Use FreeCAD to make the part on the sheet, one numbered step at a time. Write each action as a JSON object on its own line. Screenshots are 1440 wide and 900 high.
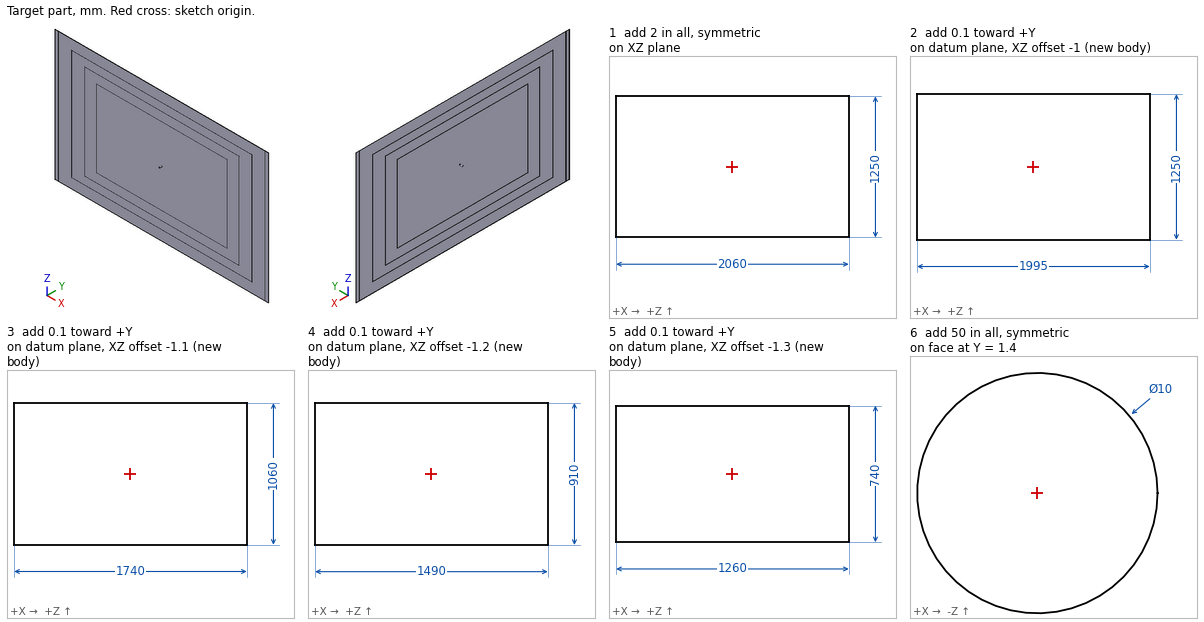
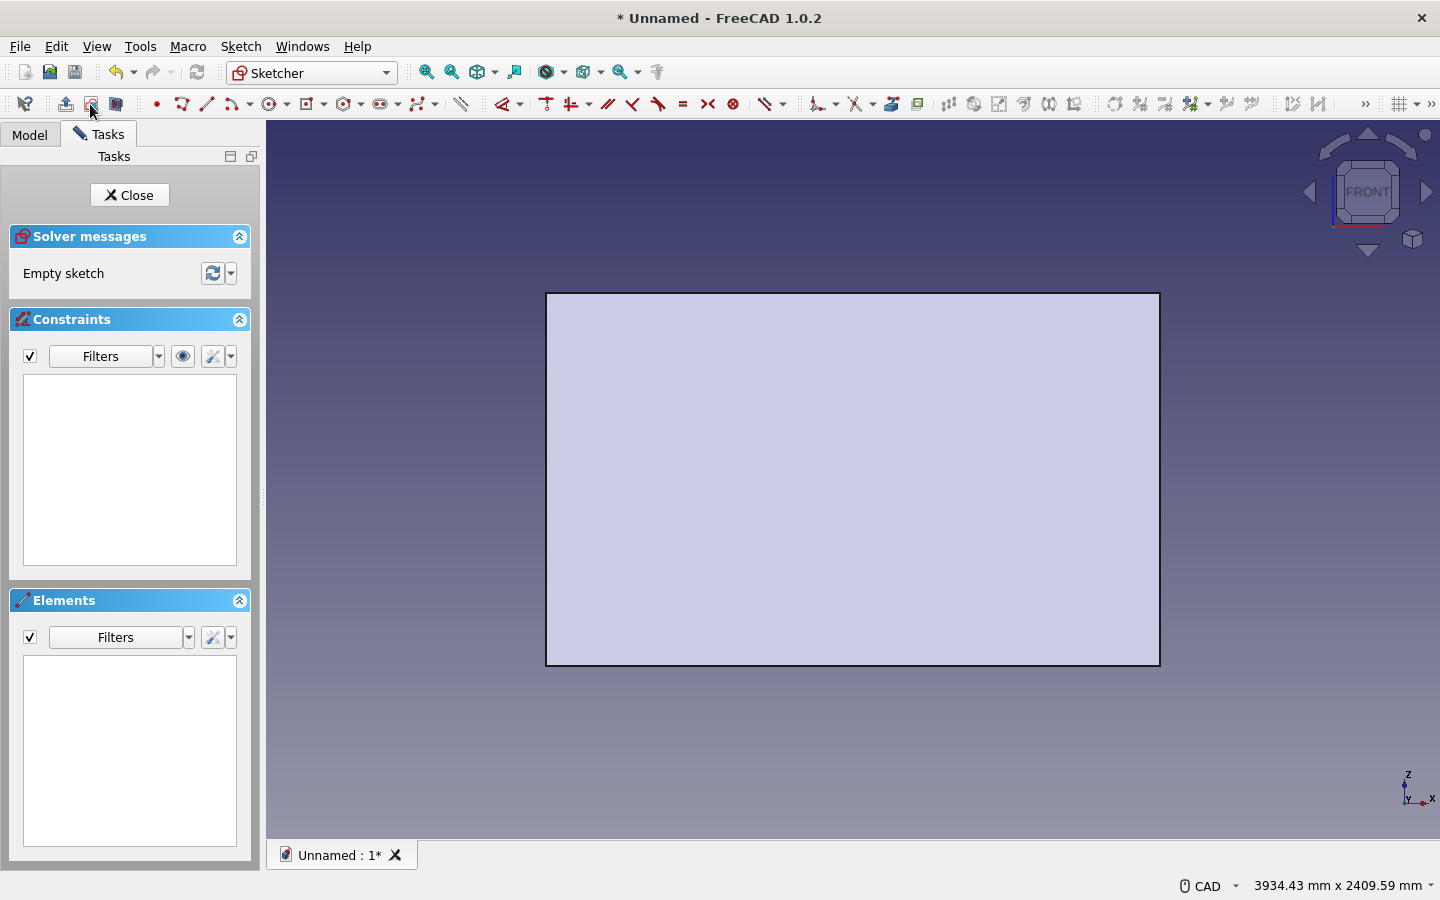
{"action": "left_click", "coordinate": [306, 104]}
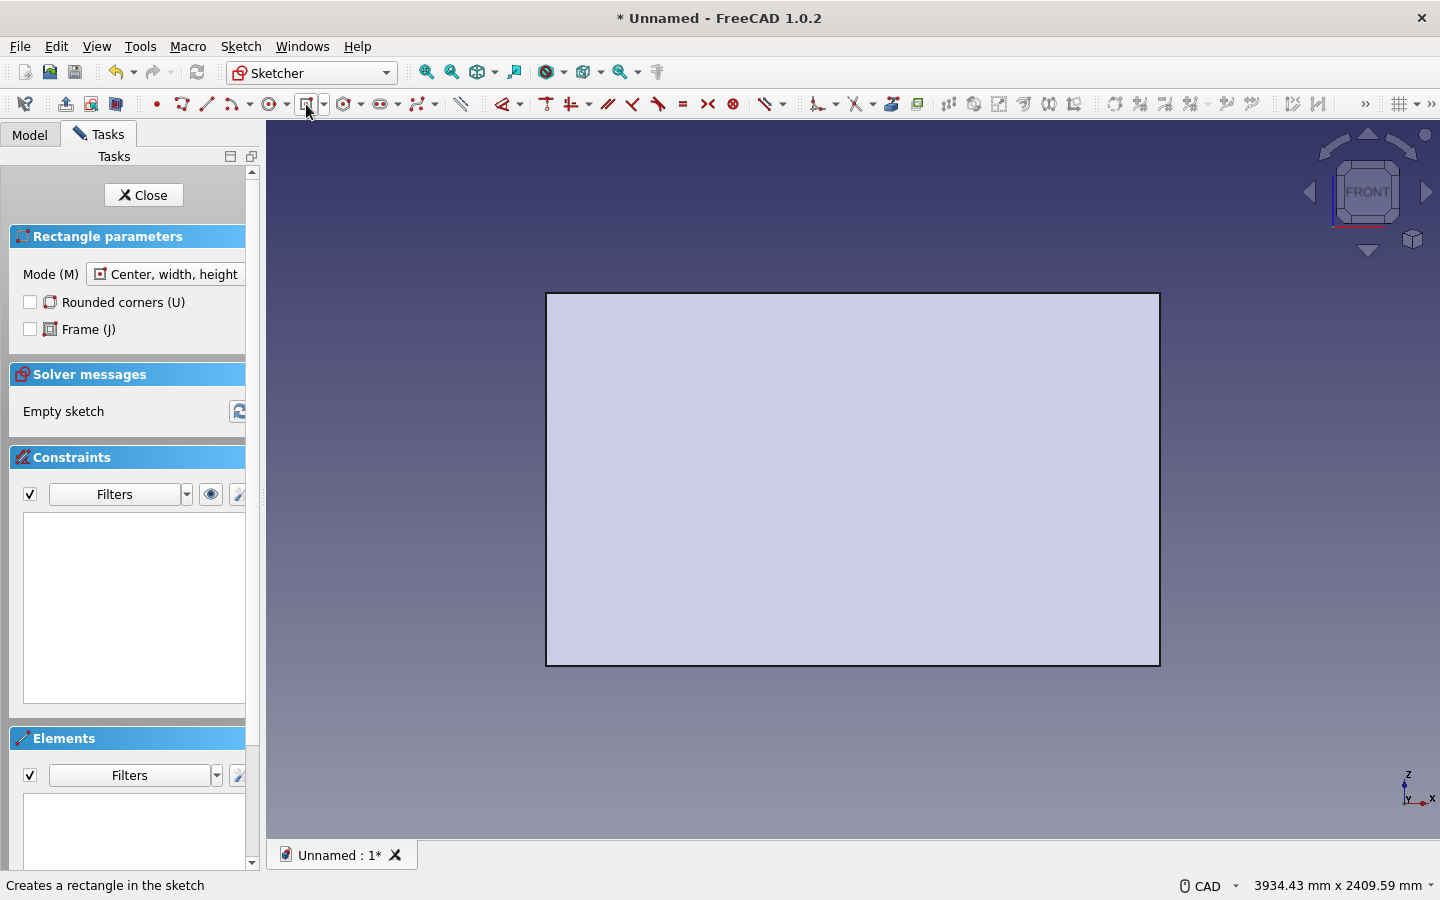
{"action": "left_click", "coordinate": [853, 480]}
{"action": "mouse_move", "coordinate": [1151, 293]}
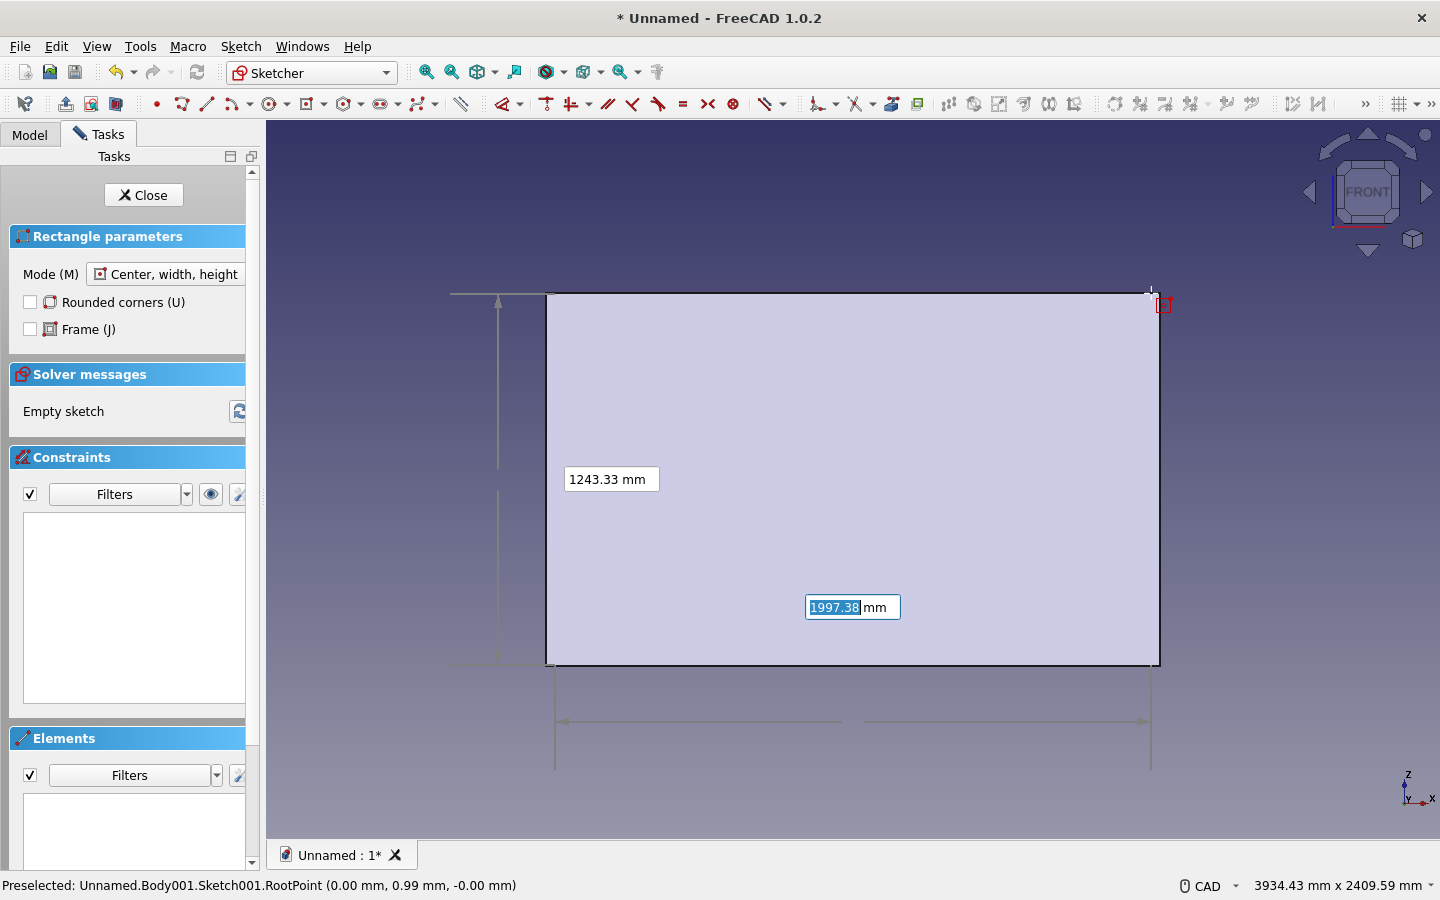
{"action": "type", "text": "1995"}
{"action": "key", "text": "Tab"}
{"action": "type", "text": "1250"}
{"action": "key", "text": "Return"}
{"action": "key", "text": "Escape"}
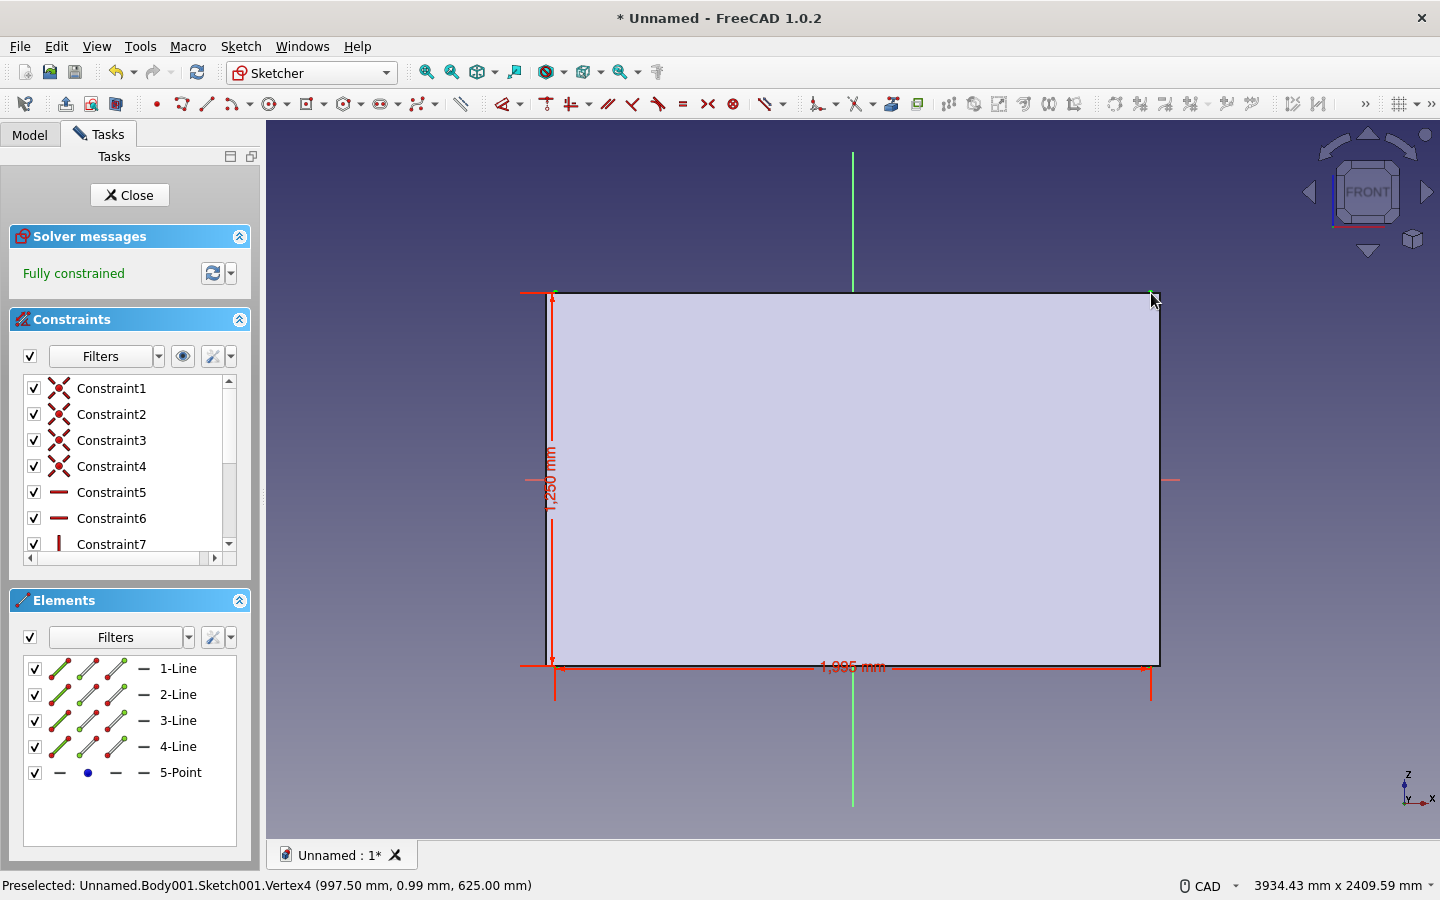
{"action": "left_click", "coordinate": [130, 195]}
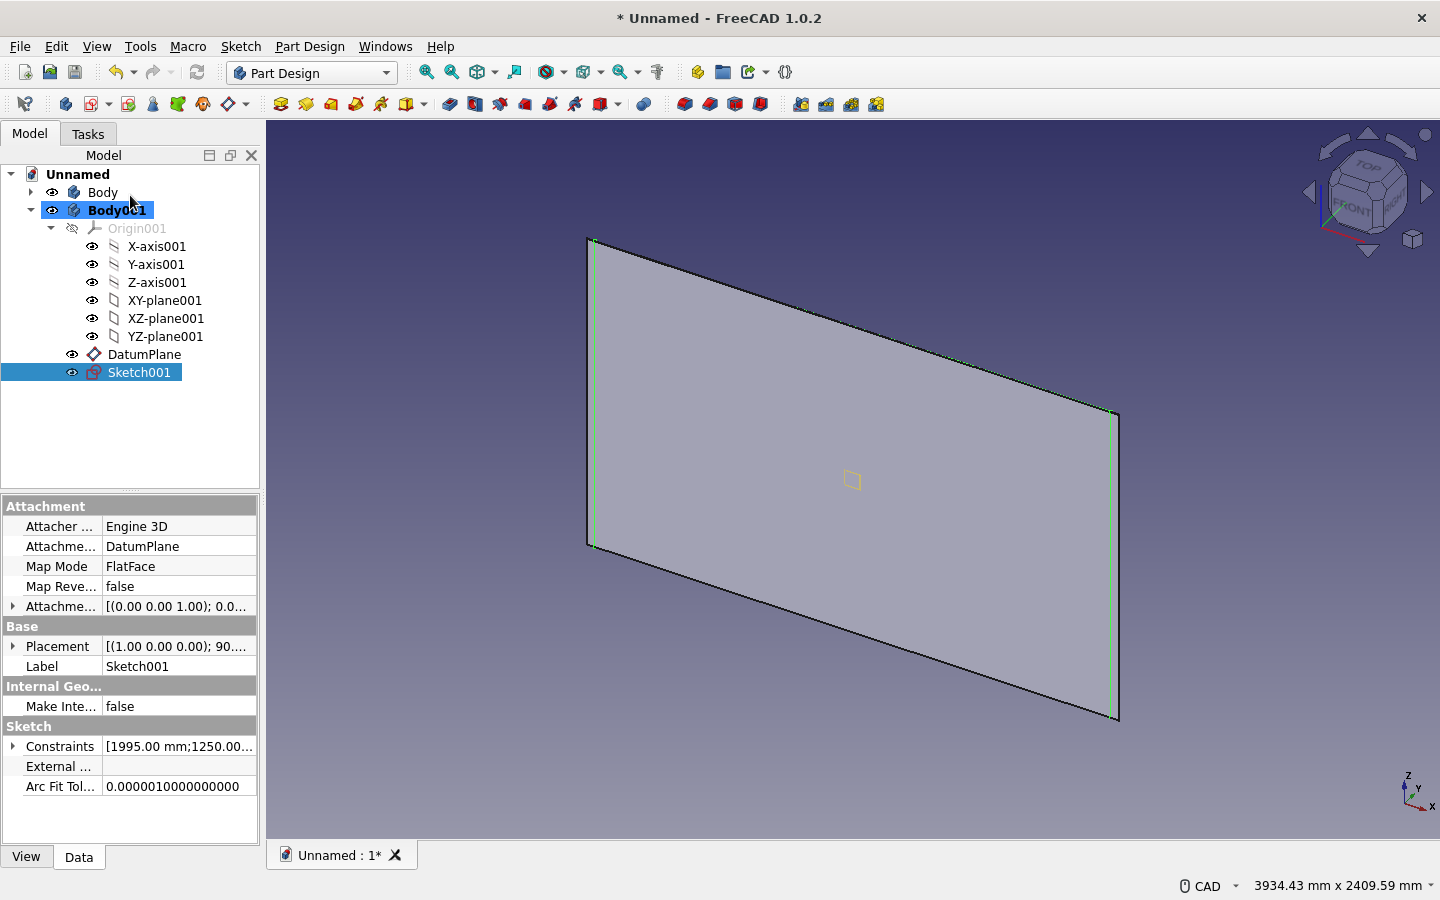
{"action": "left_click", "coordinate": [281, 104]}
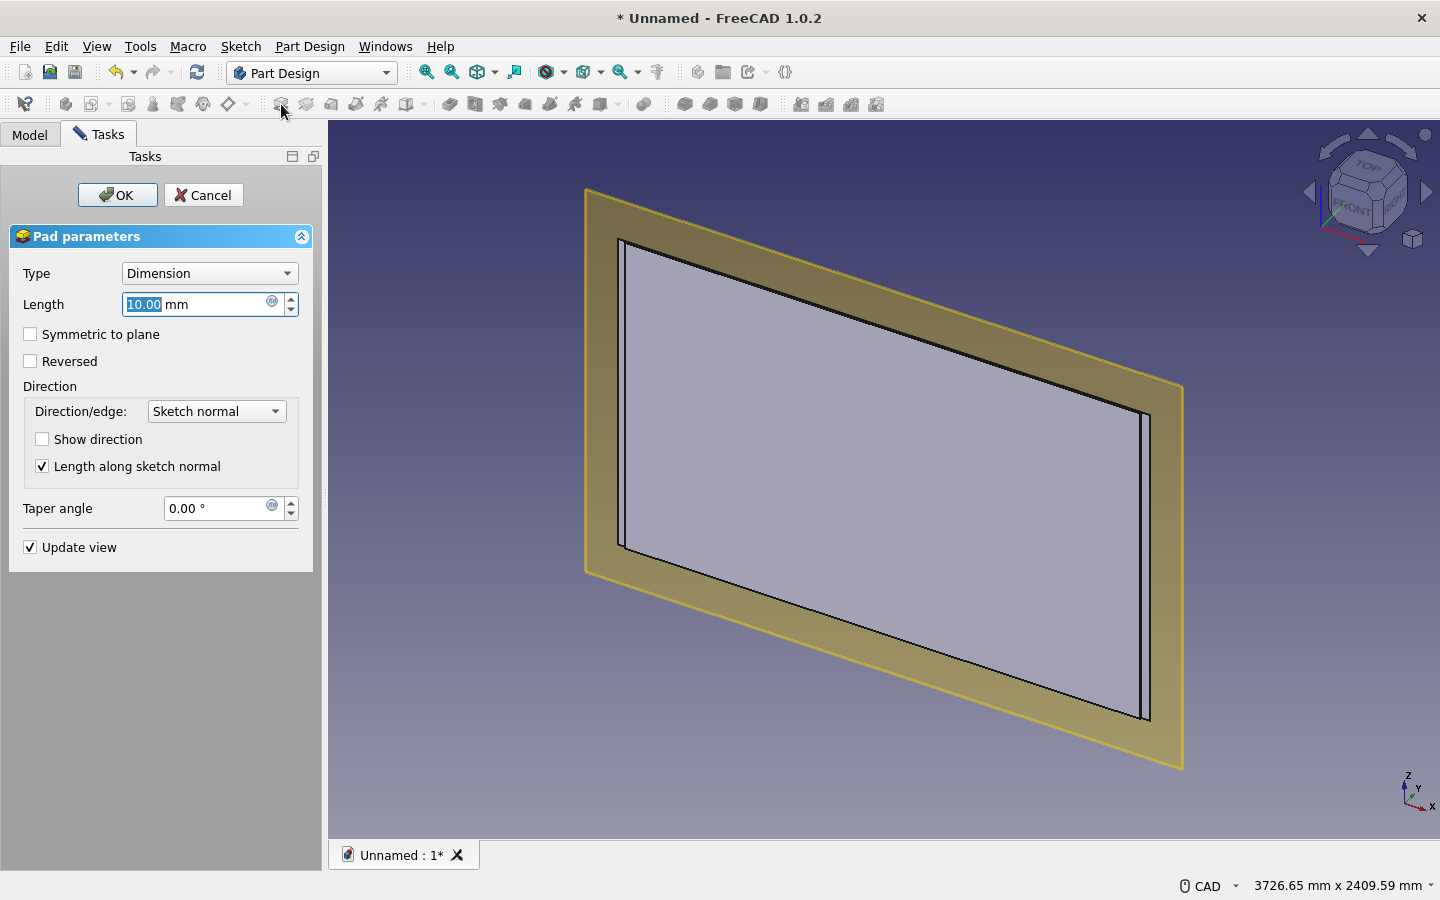
{"action": "type", "text": "0.1"}
{"action": "key", "text": "Tab"}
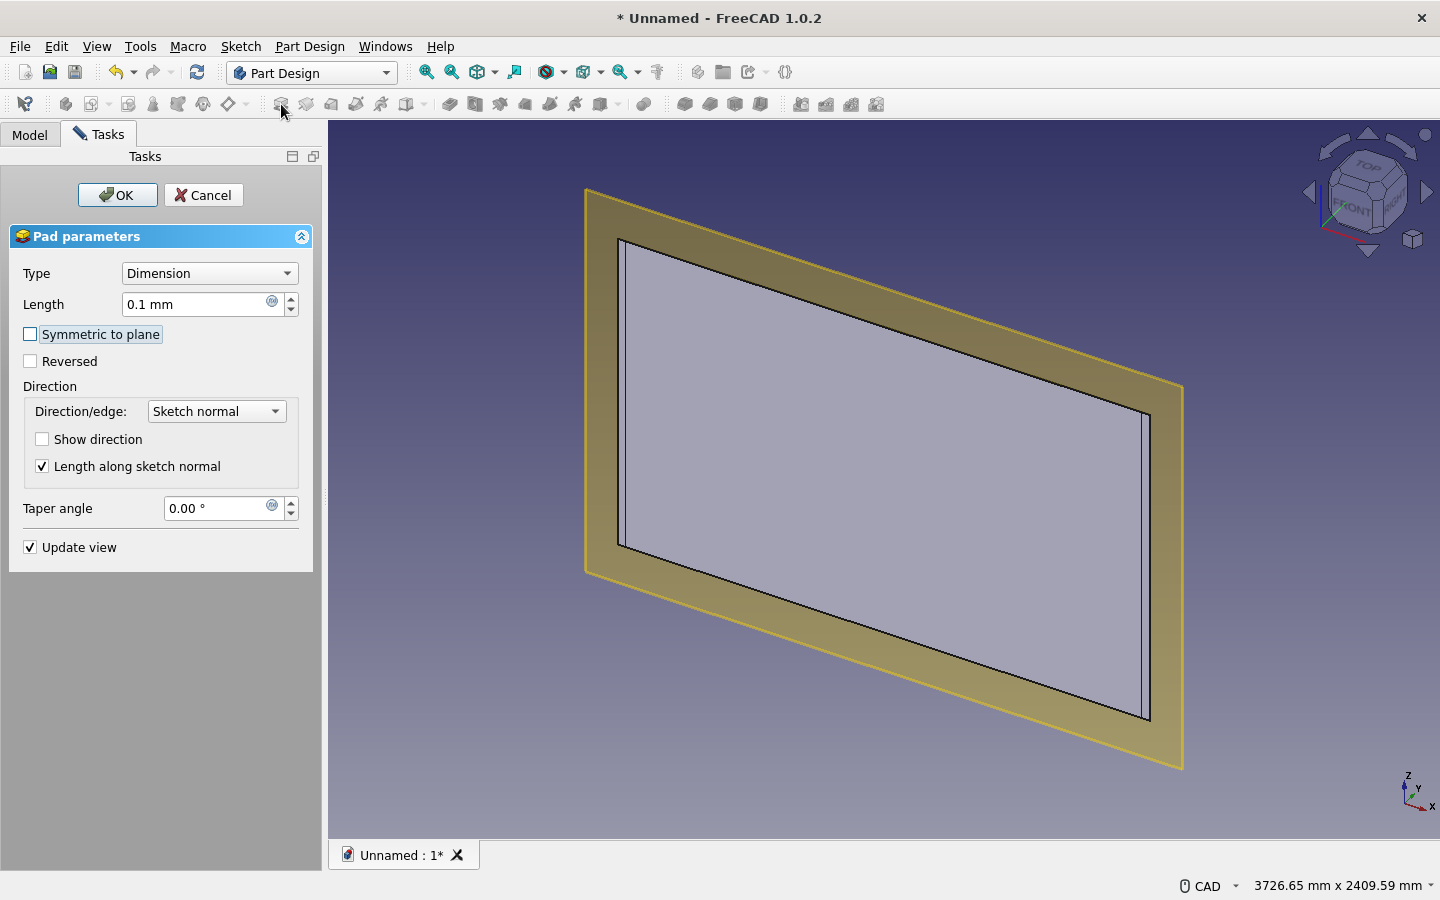
{"action": "left_click", "coordinate": [31, 361]}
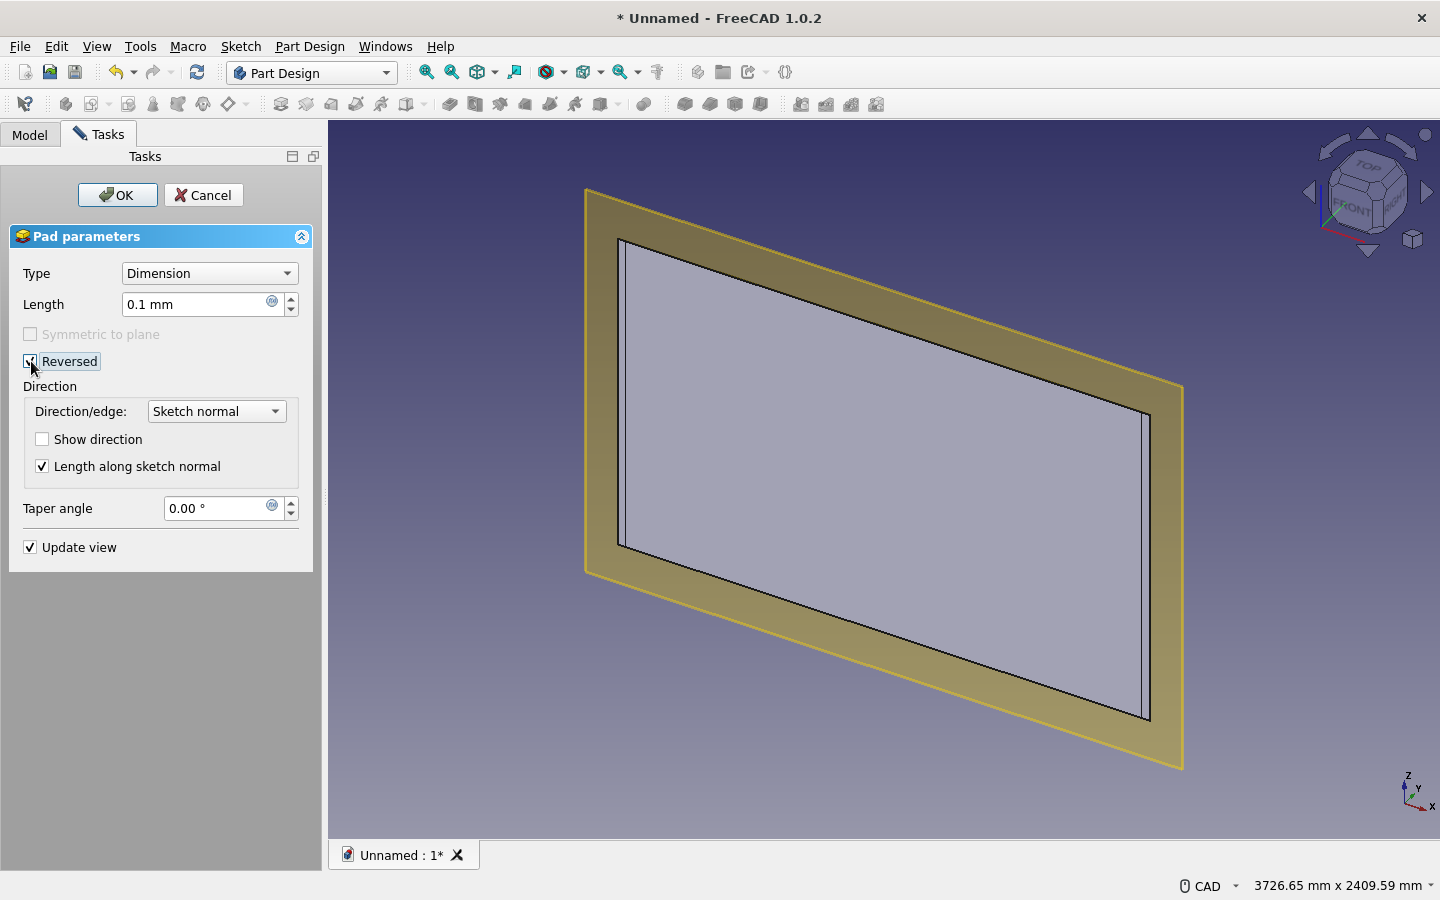
{"action": "left_click", "coordinate": [118, 195]}